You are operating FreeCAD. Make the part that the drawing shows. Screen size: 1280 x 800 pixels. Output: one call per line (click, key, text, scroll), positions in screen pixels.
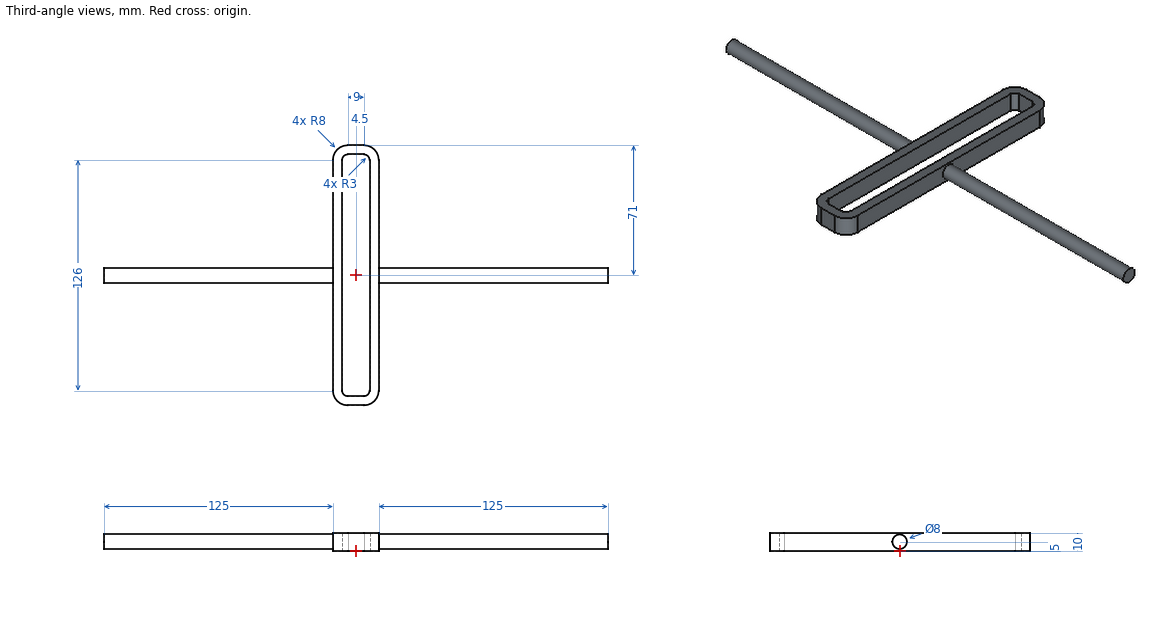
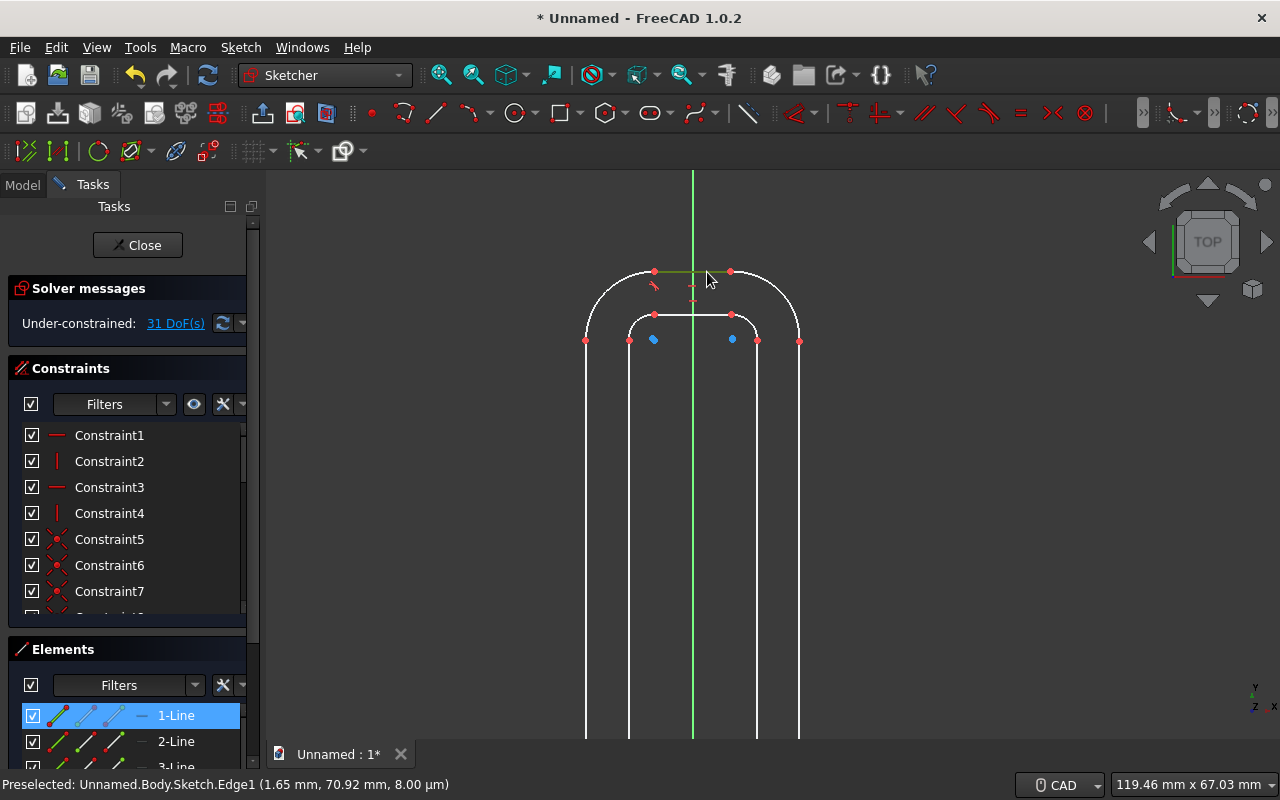
click(793, 310)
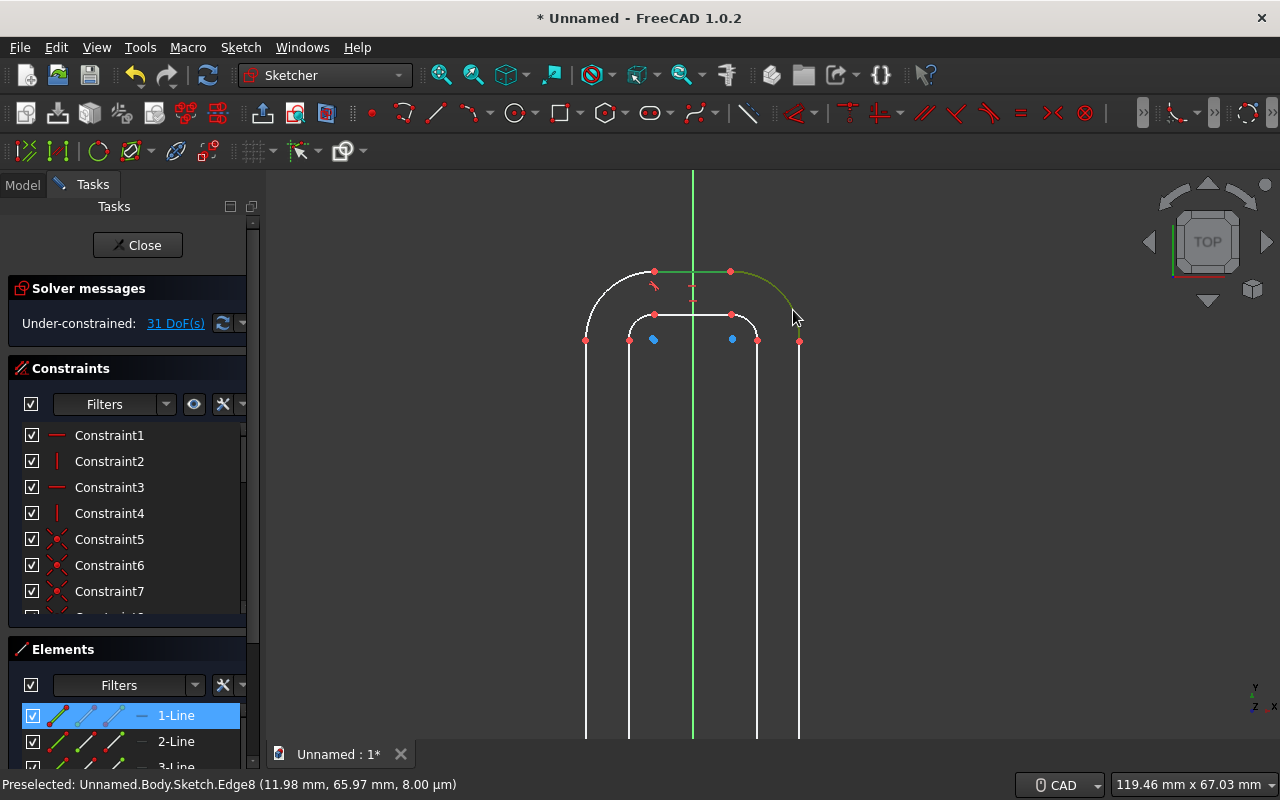
click(990, 114)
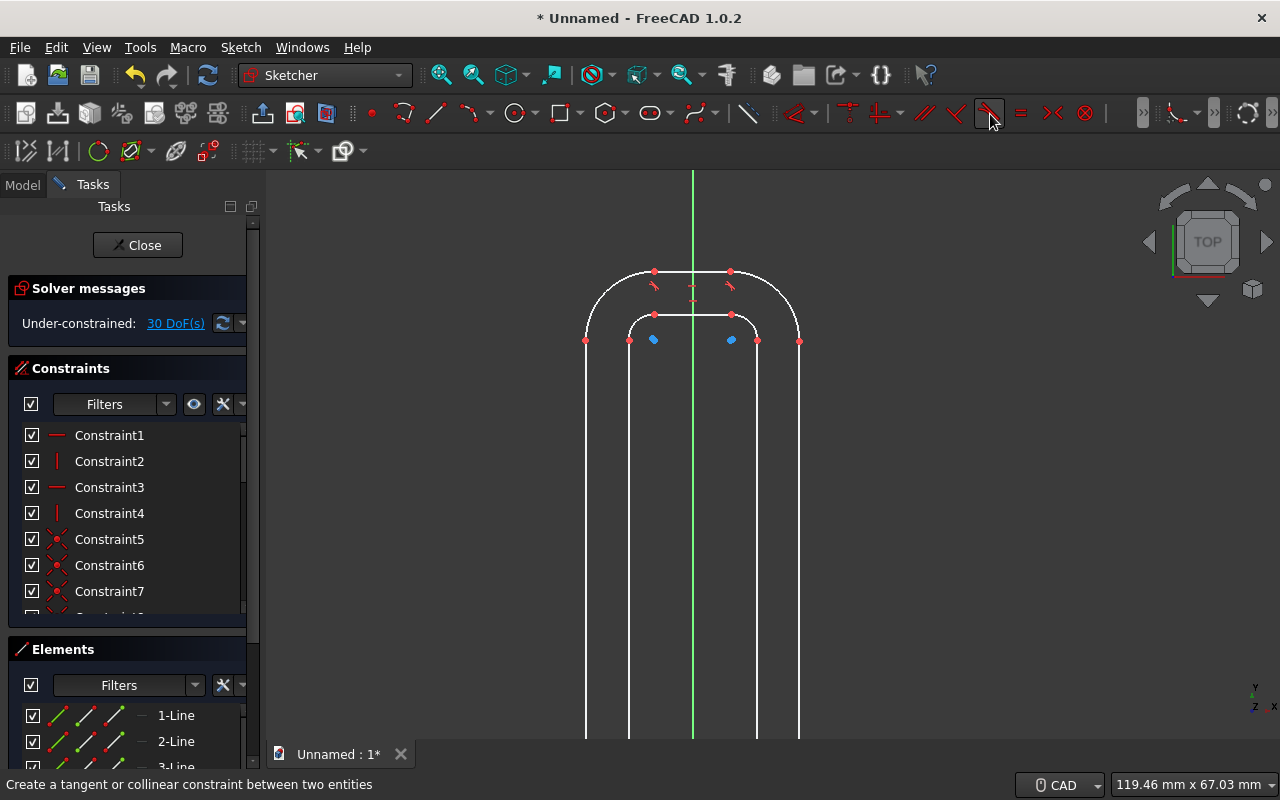
click(586, 661)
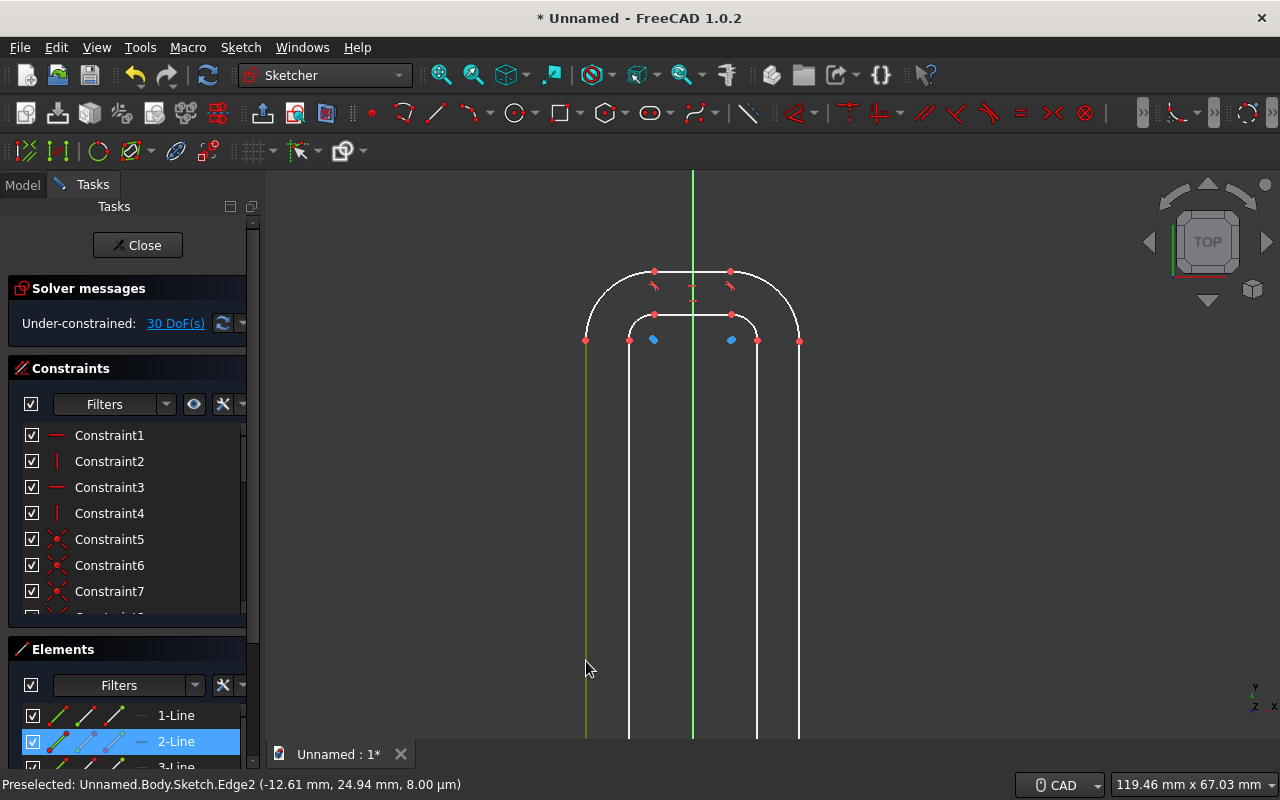
click(623, 279)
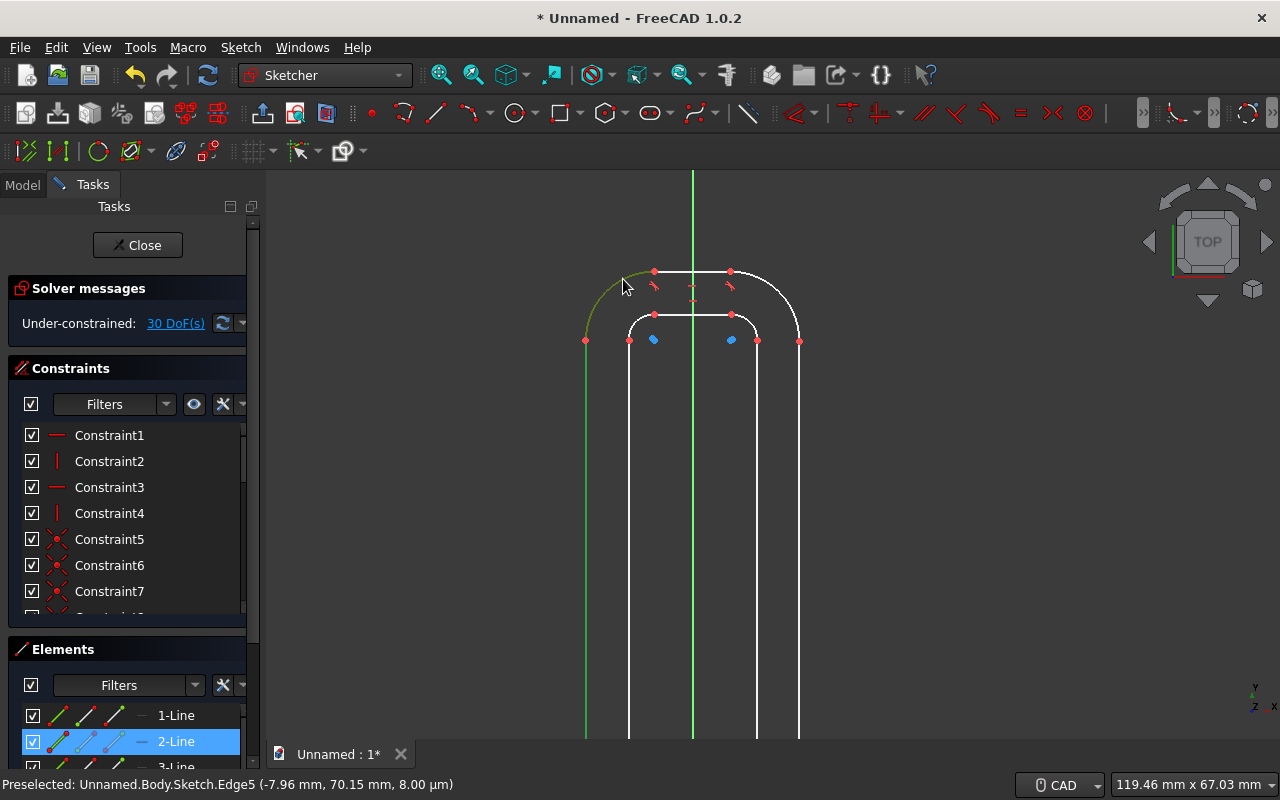
click(990, 114)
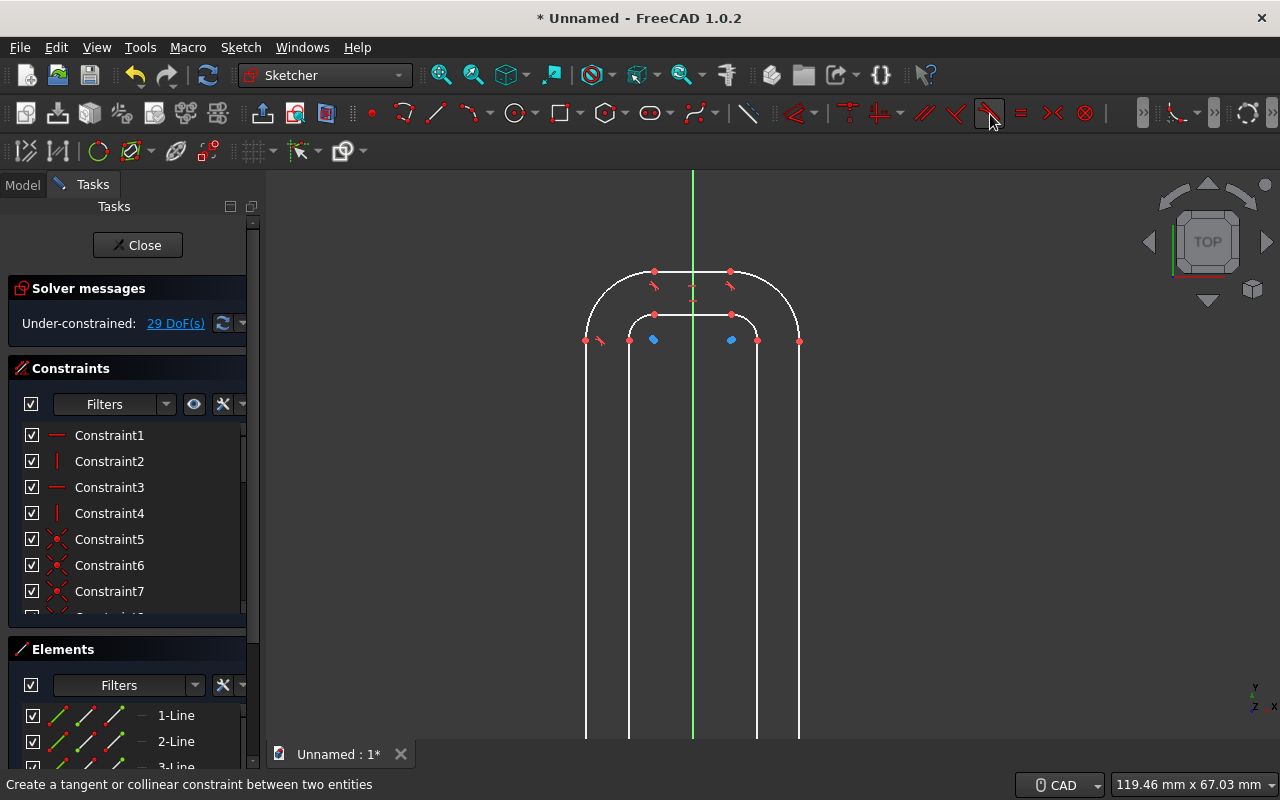
click(586, 661)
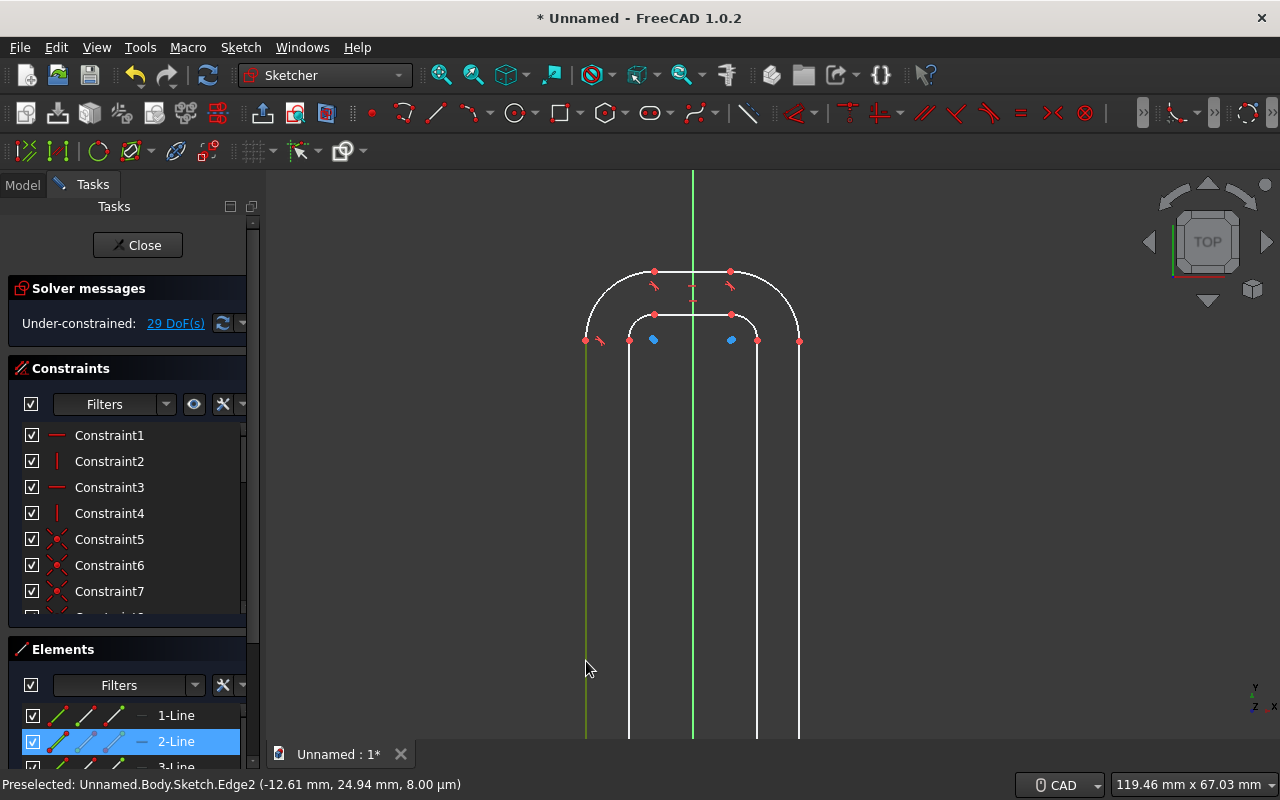
scroll(709, 274, down, 6)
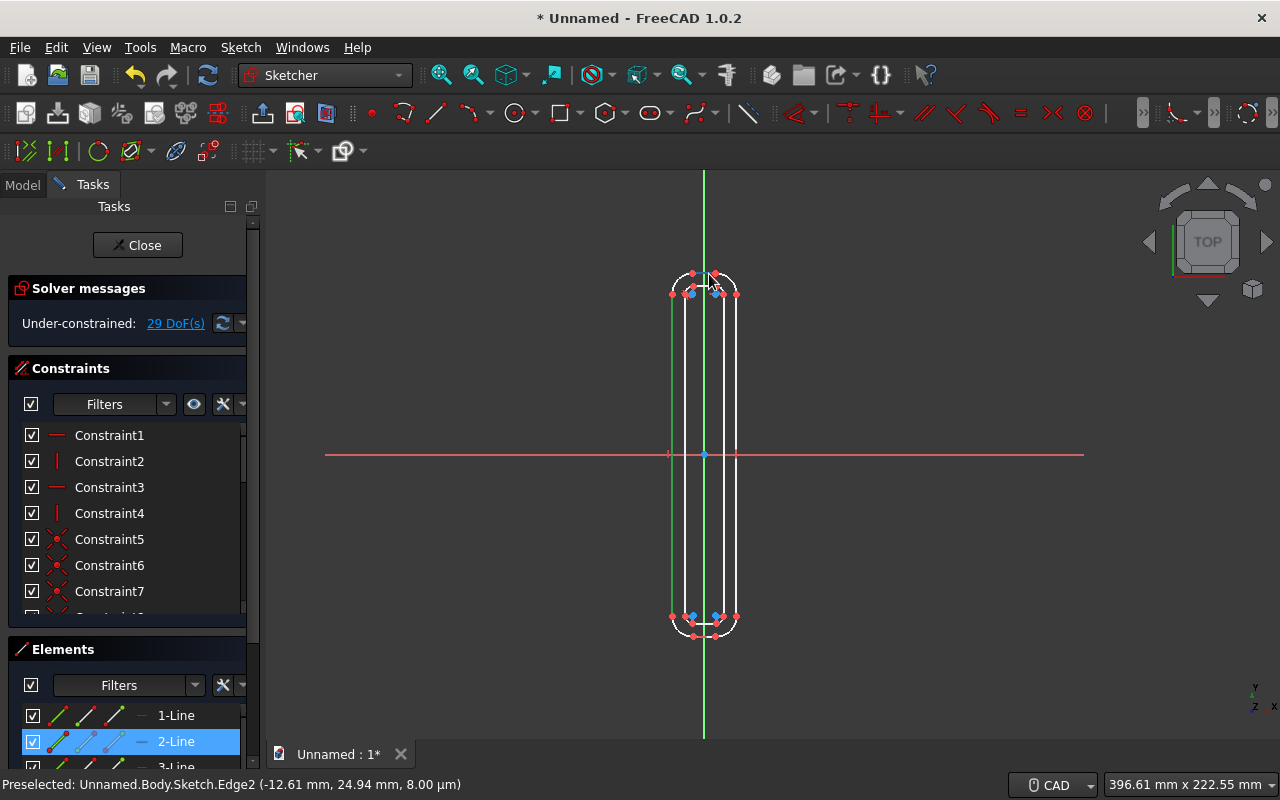
scroll(675, 626, up, 2)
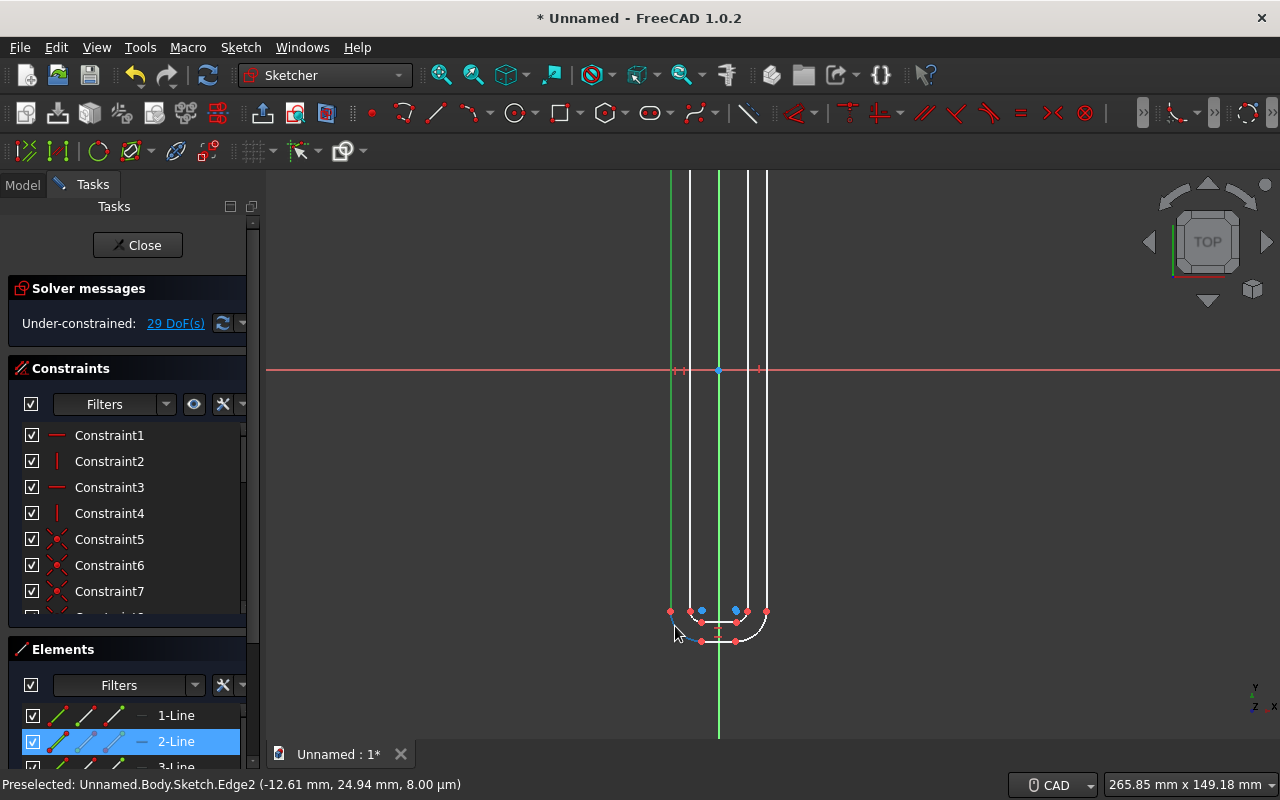
click(674, 625)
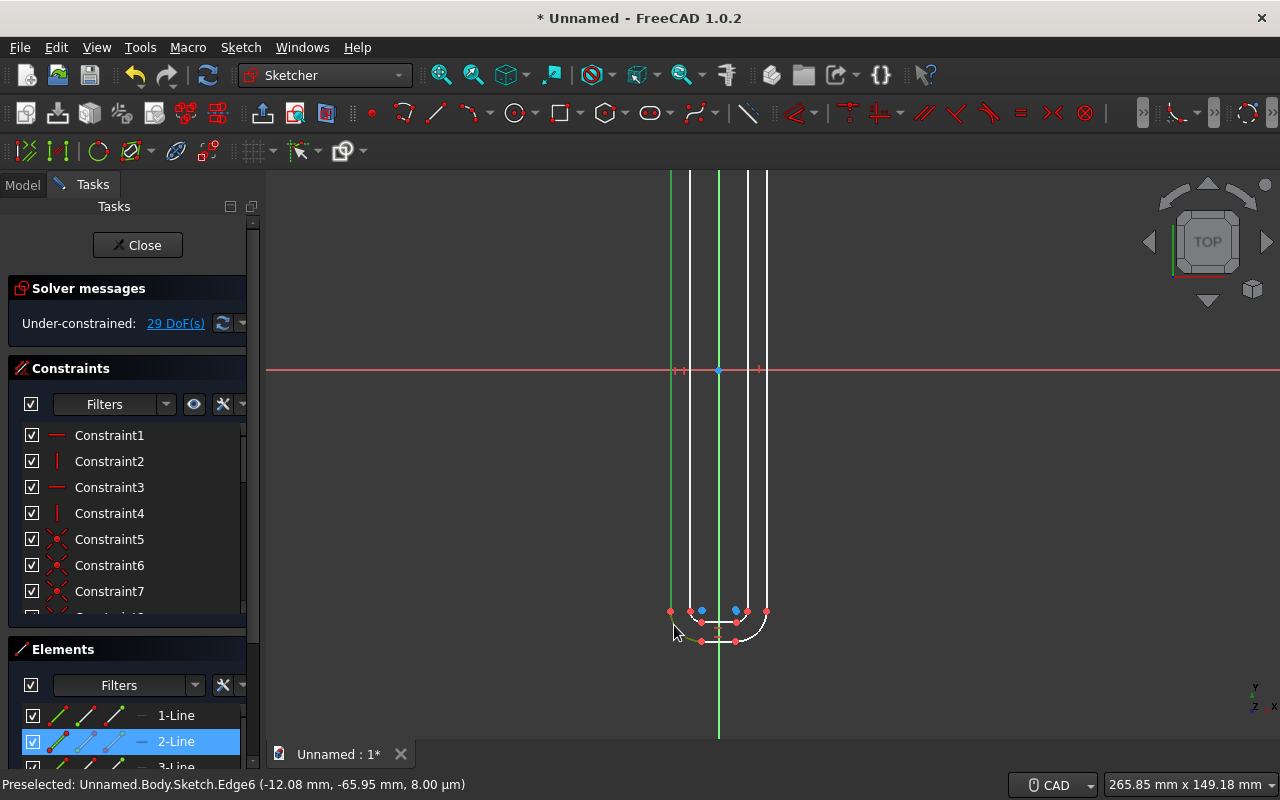
click(990, 114)